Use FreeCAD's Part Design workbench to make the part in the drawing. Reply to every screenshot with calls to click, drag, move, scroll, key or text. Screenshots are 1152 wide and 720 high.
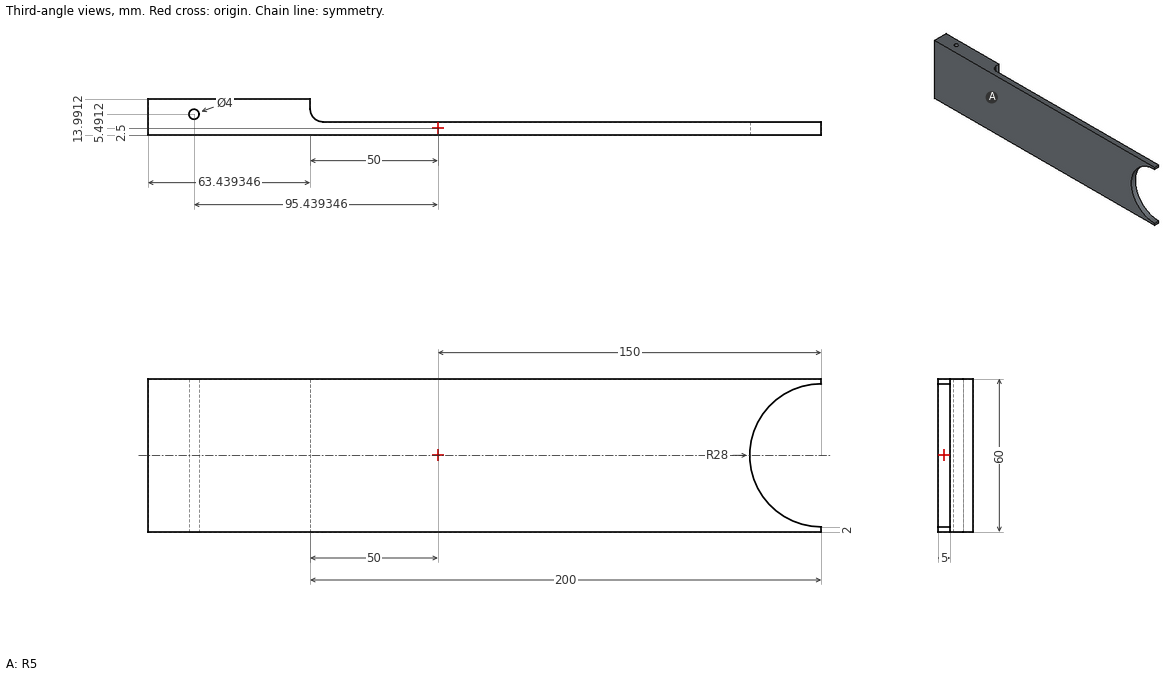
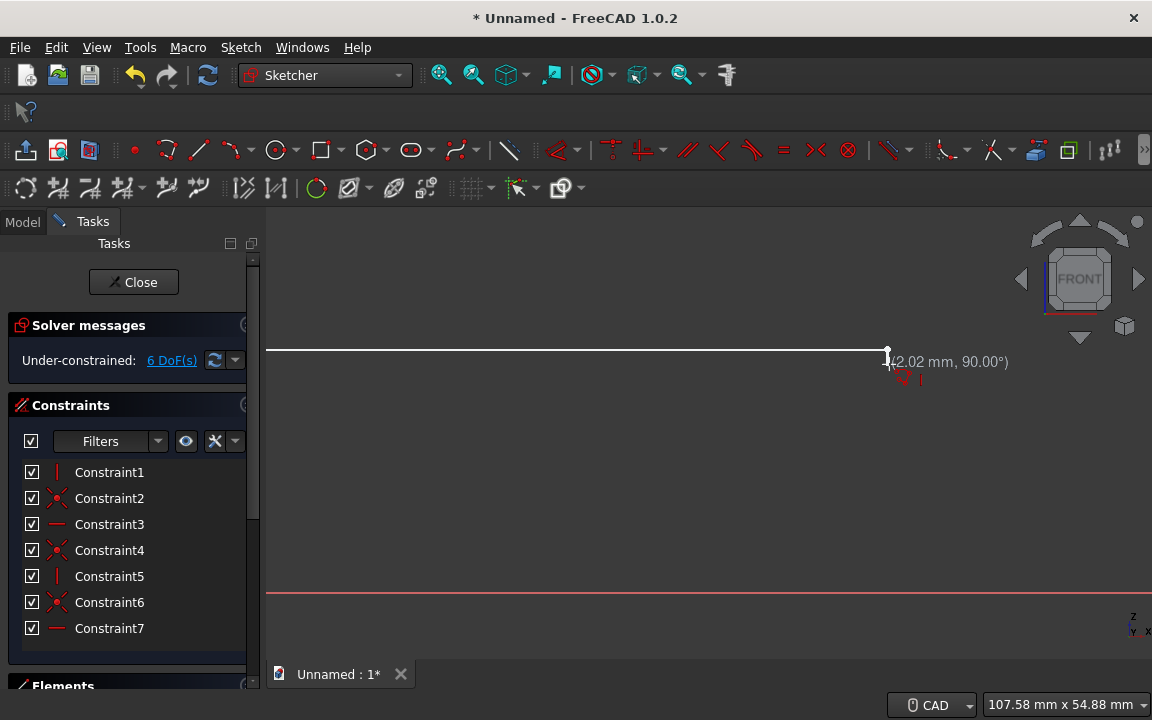
click(887, 362)
right_click(887, 362)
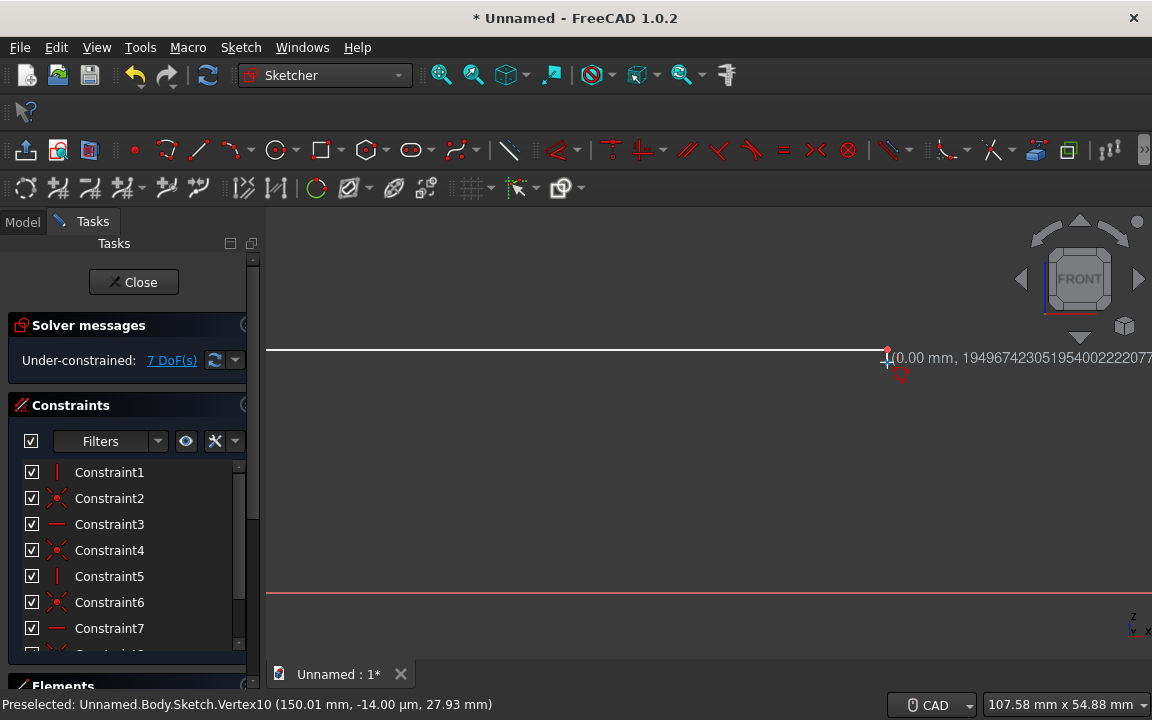
click(232, 150)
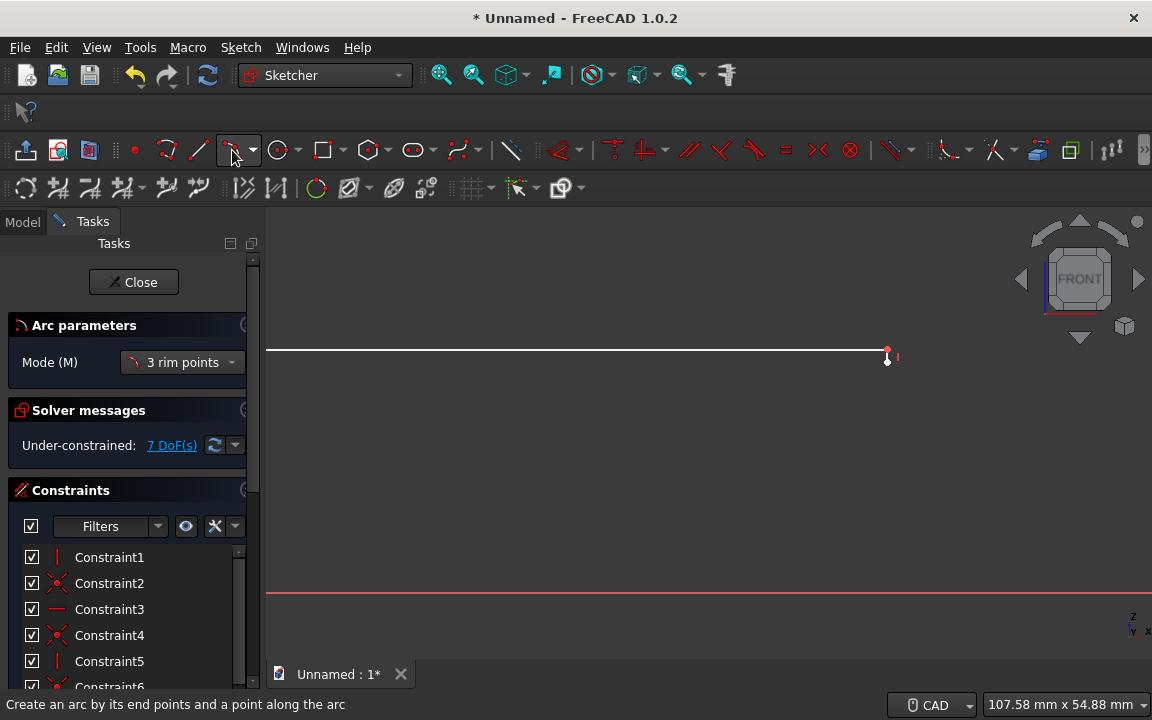
scroll(887, 362, up, 4)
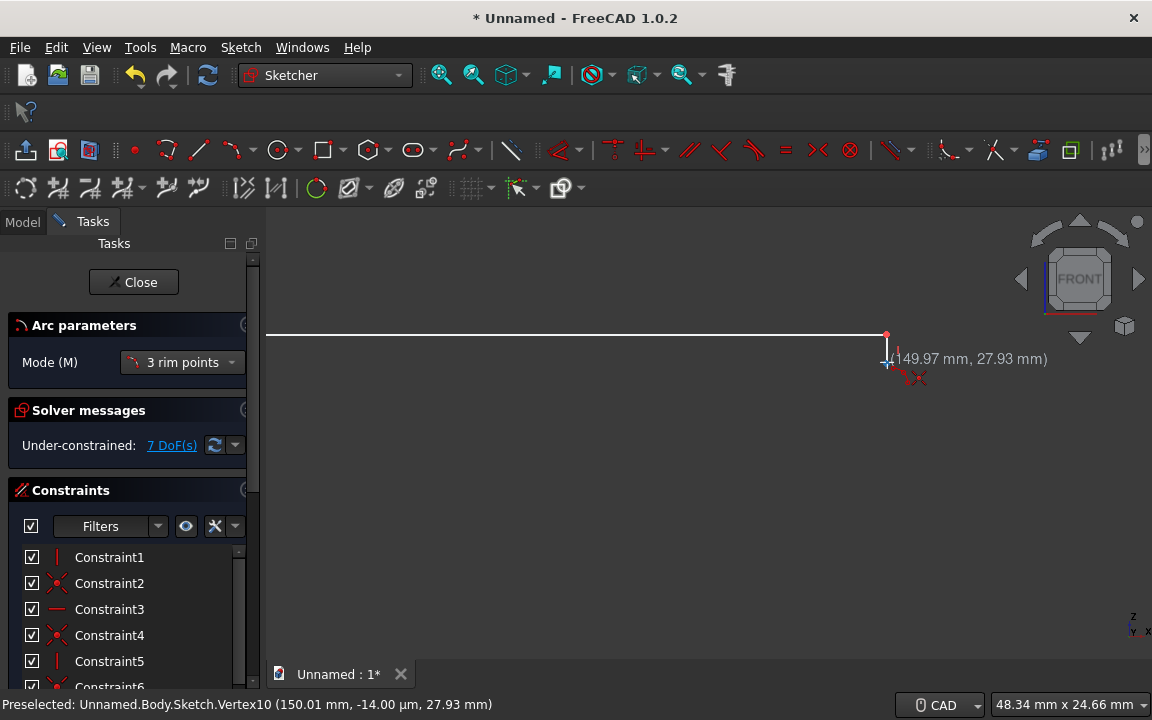
click(887, 364)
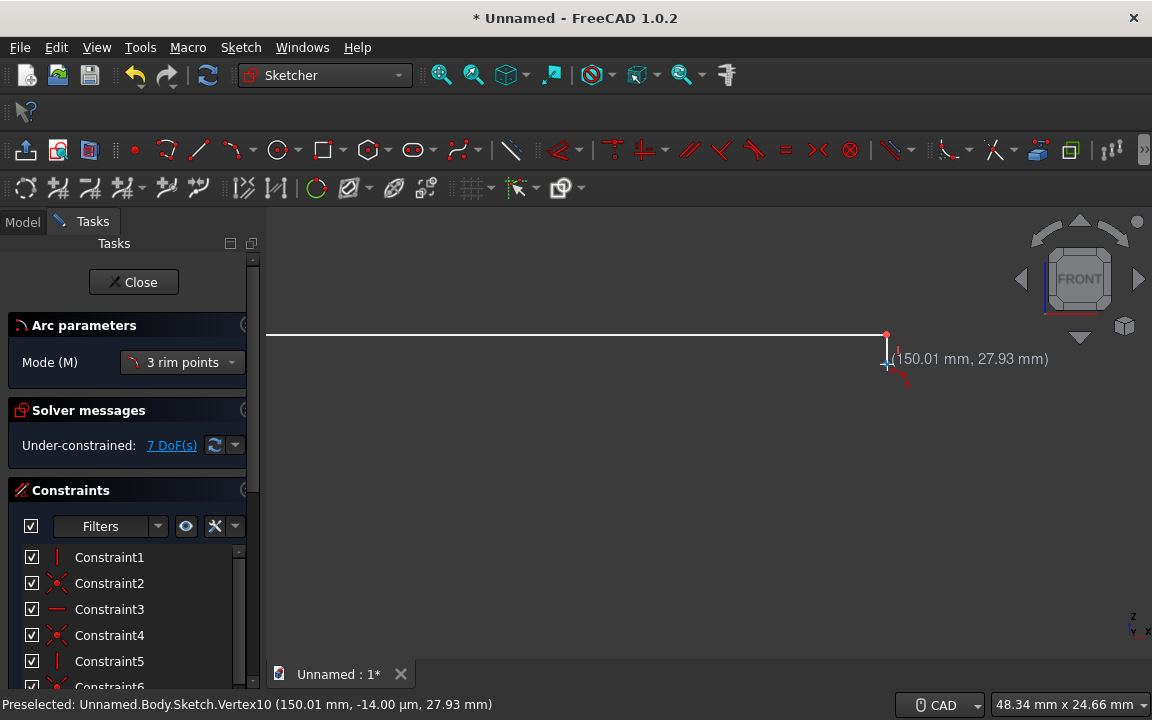
scroll(889, 364, down, 10)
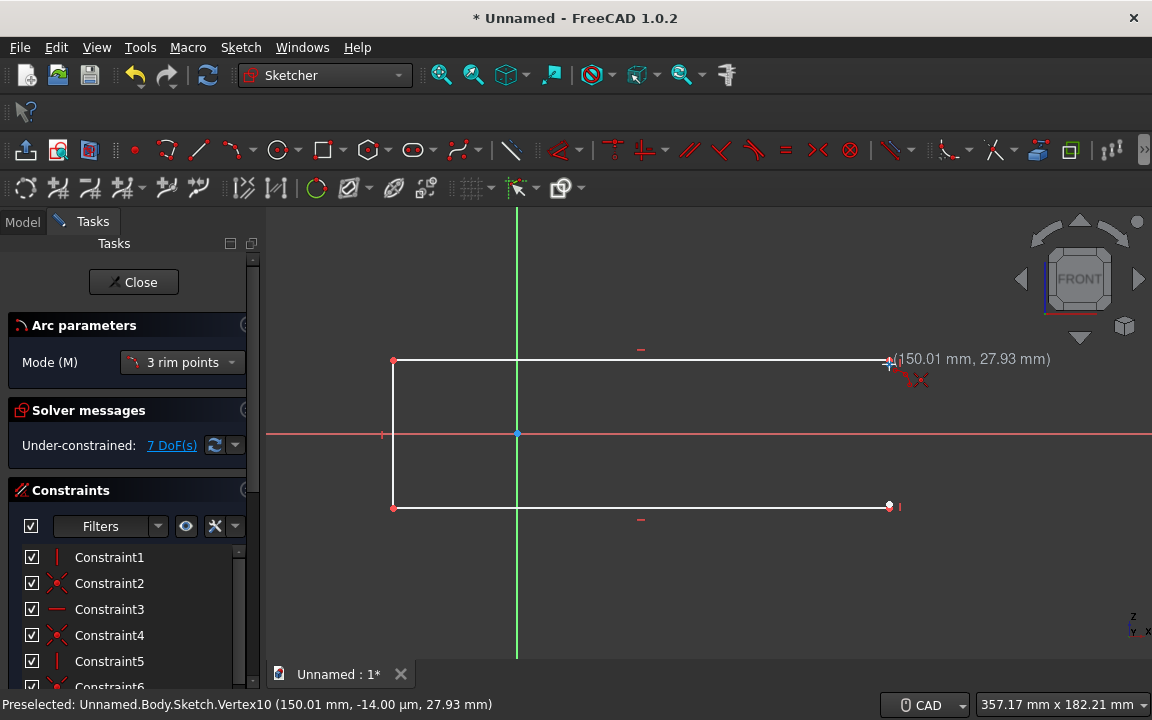
scroll(889, 503, up, 10)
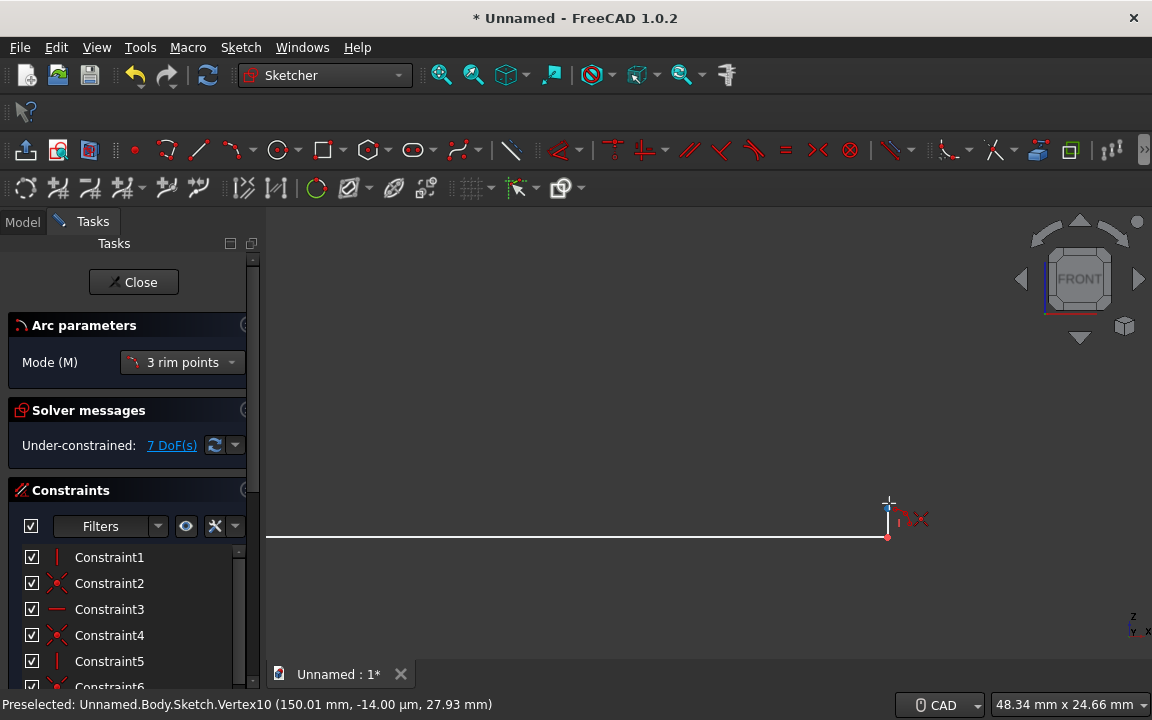
click(888, 509)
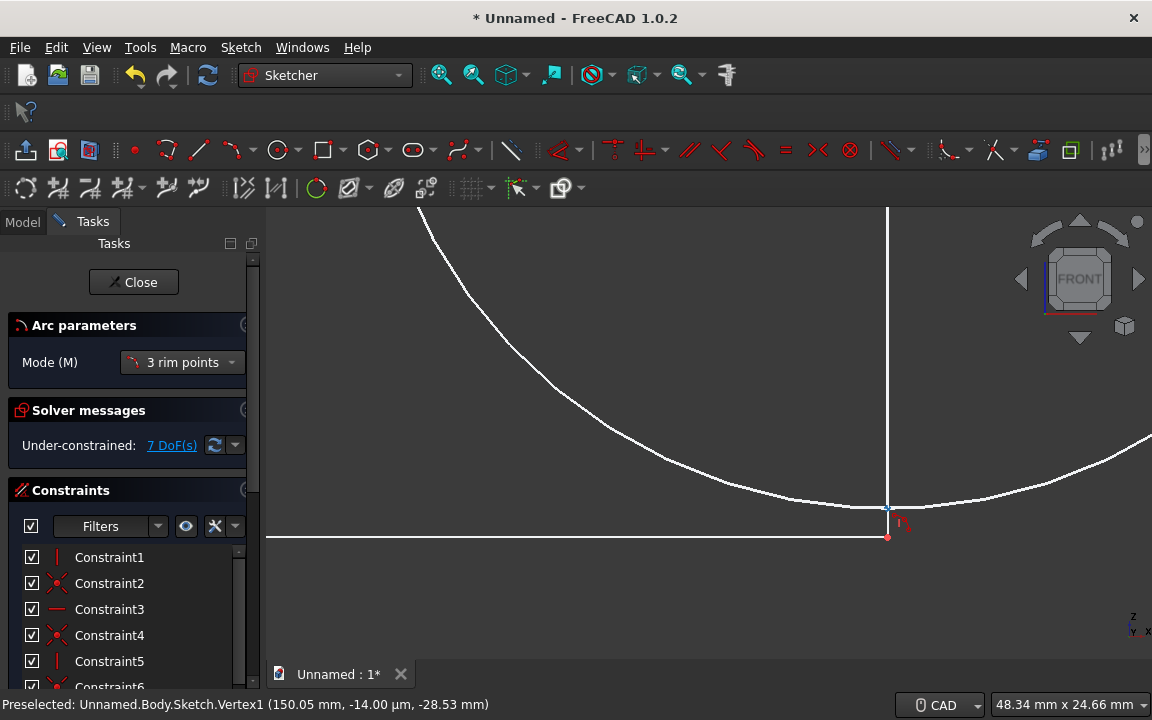
scroll(889, 503, down, 10)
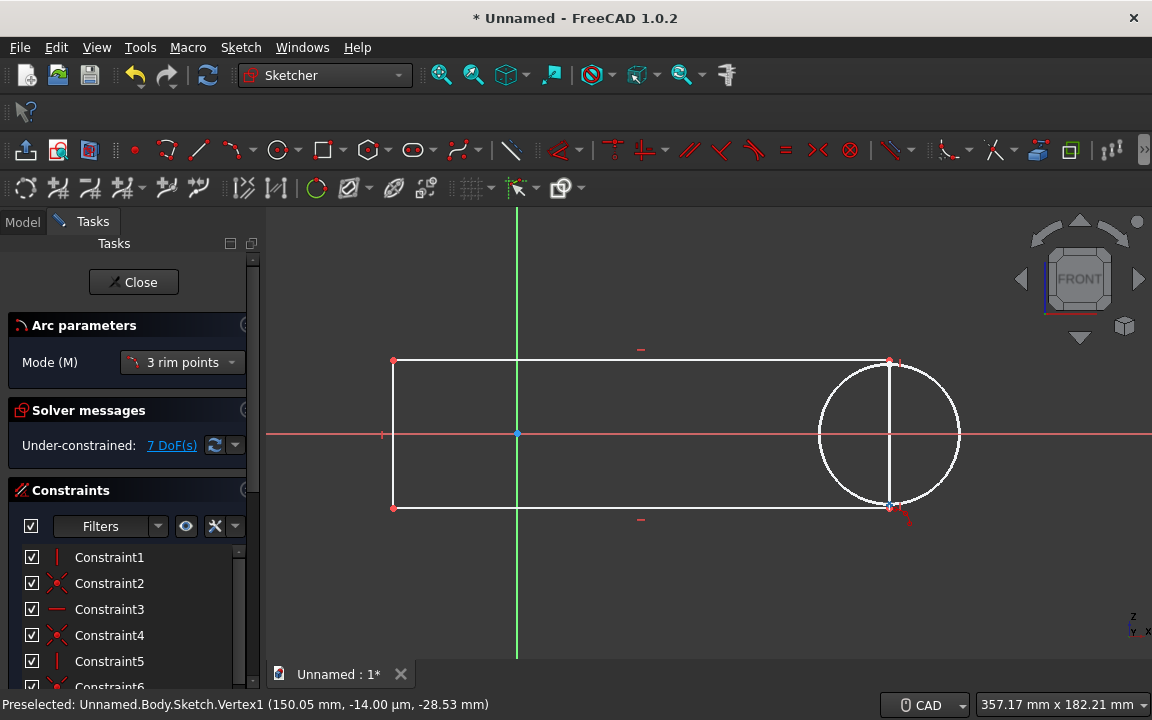
click(823, 412)
key(Escape)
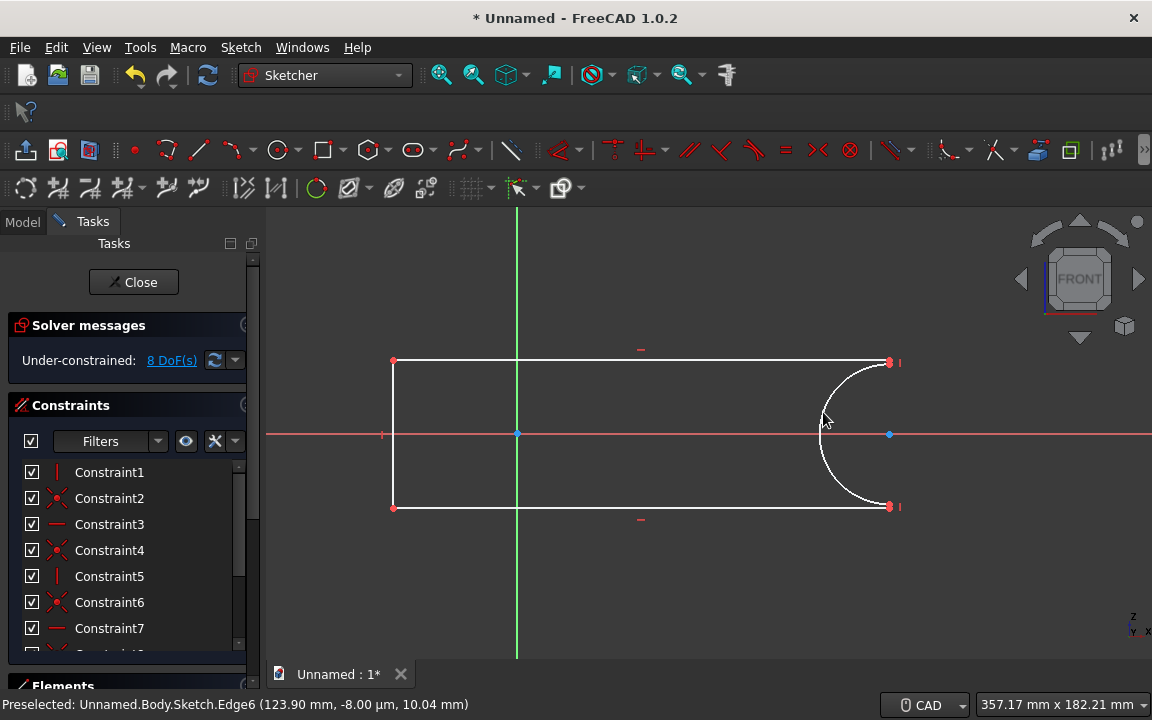
click(890, 434)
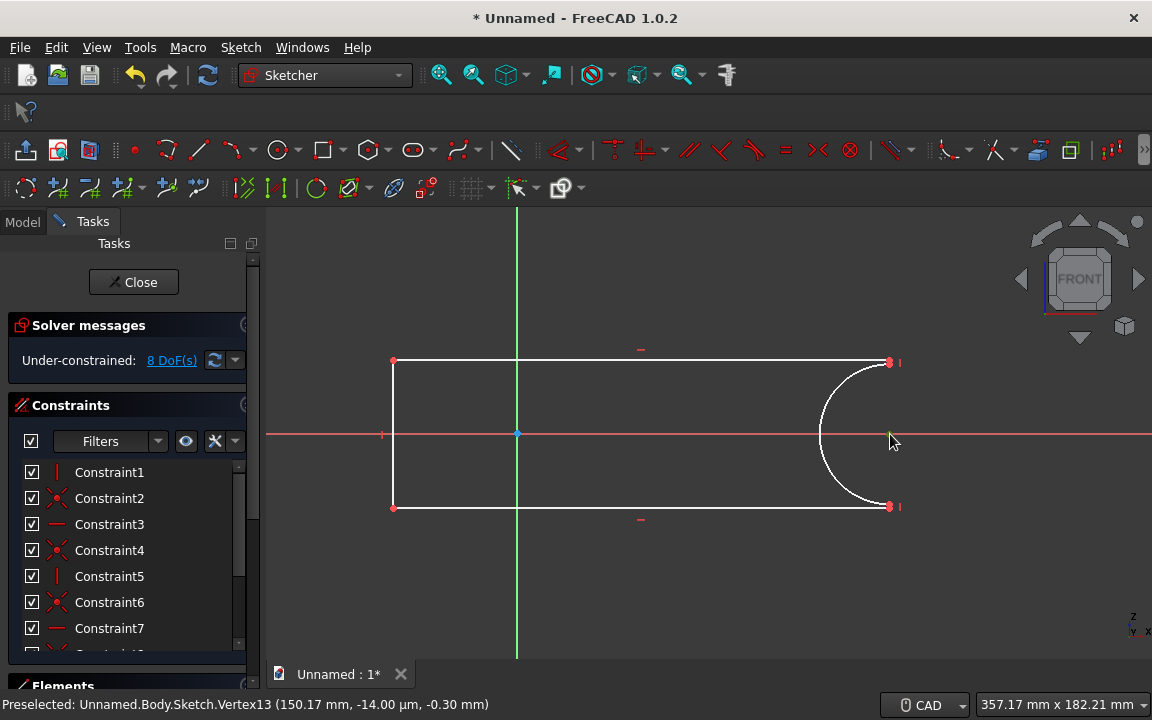
click(344, 434)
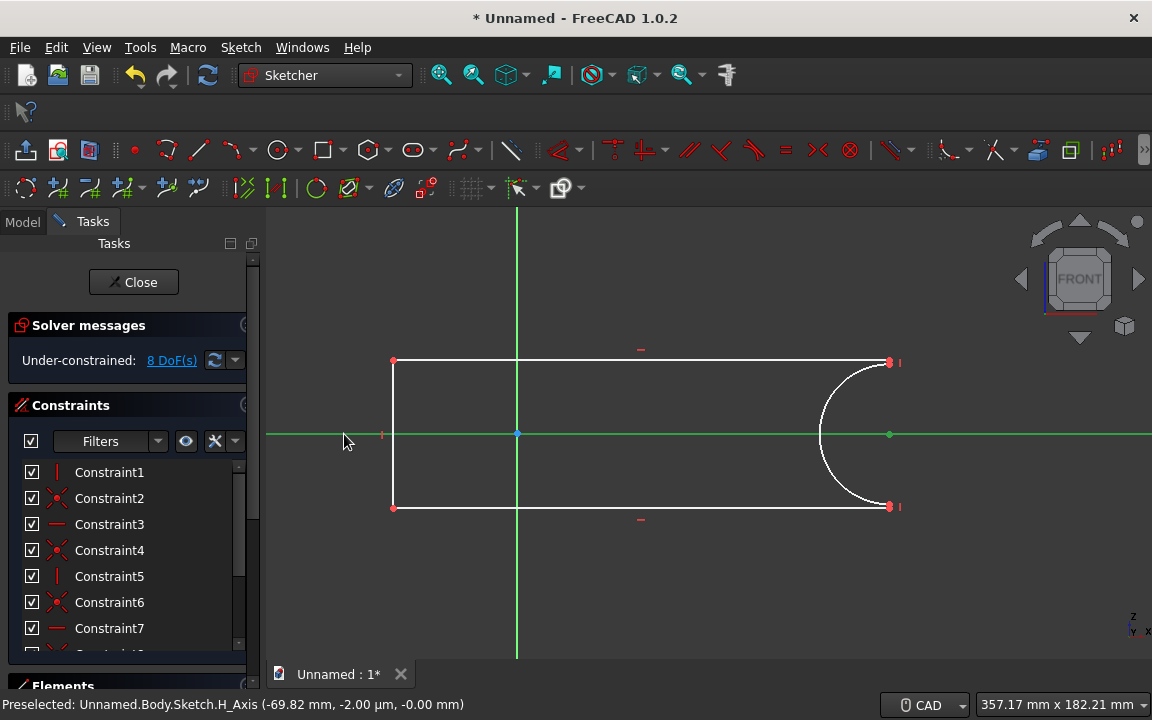
key(c)